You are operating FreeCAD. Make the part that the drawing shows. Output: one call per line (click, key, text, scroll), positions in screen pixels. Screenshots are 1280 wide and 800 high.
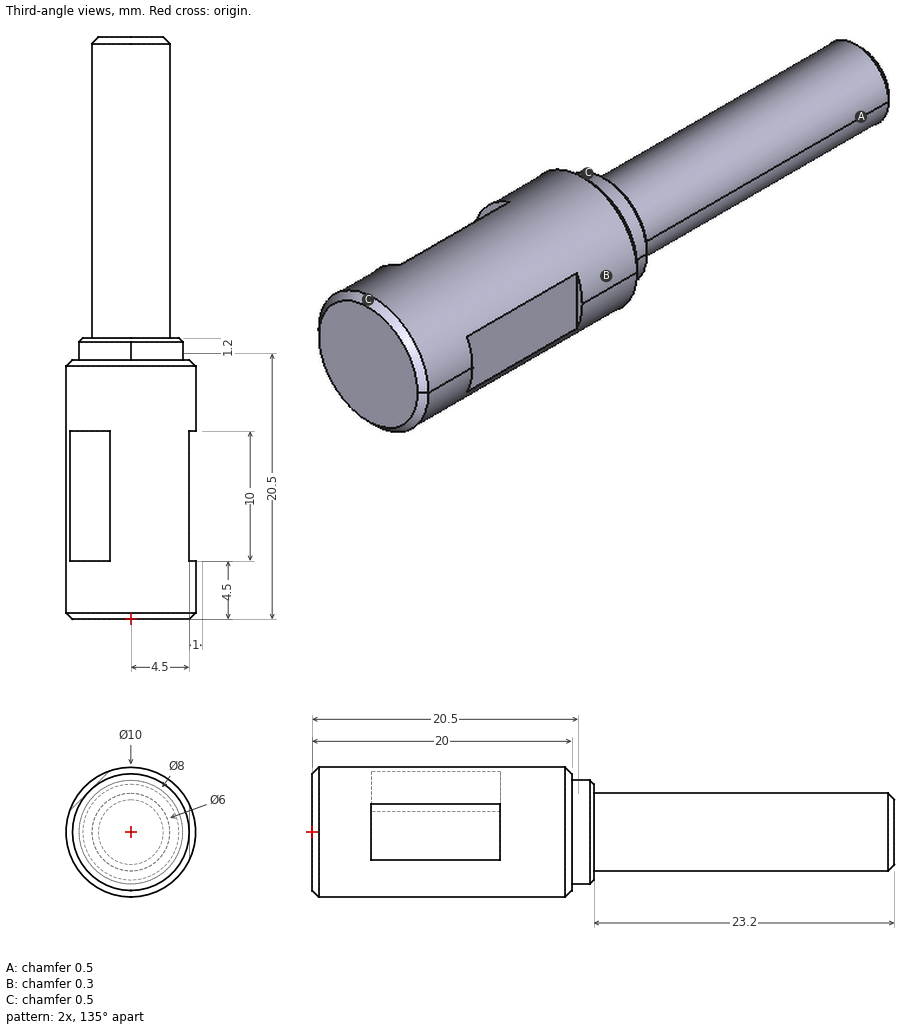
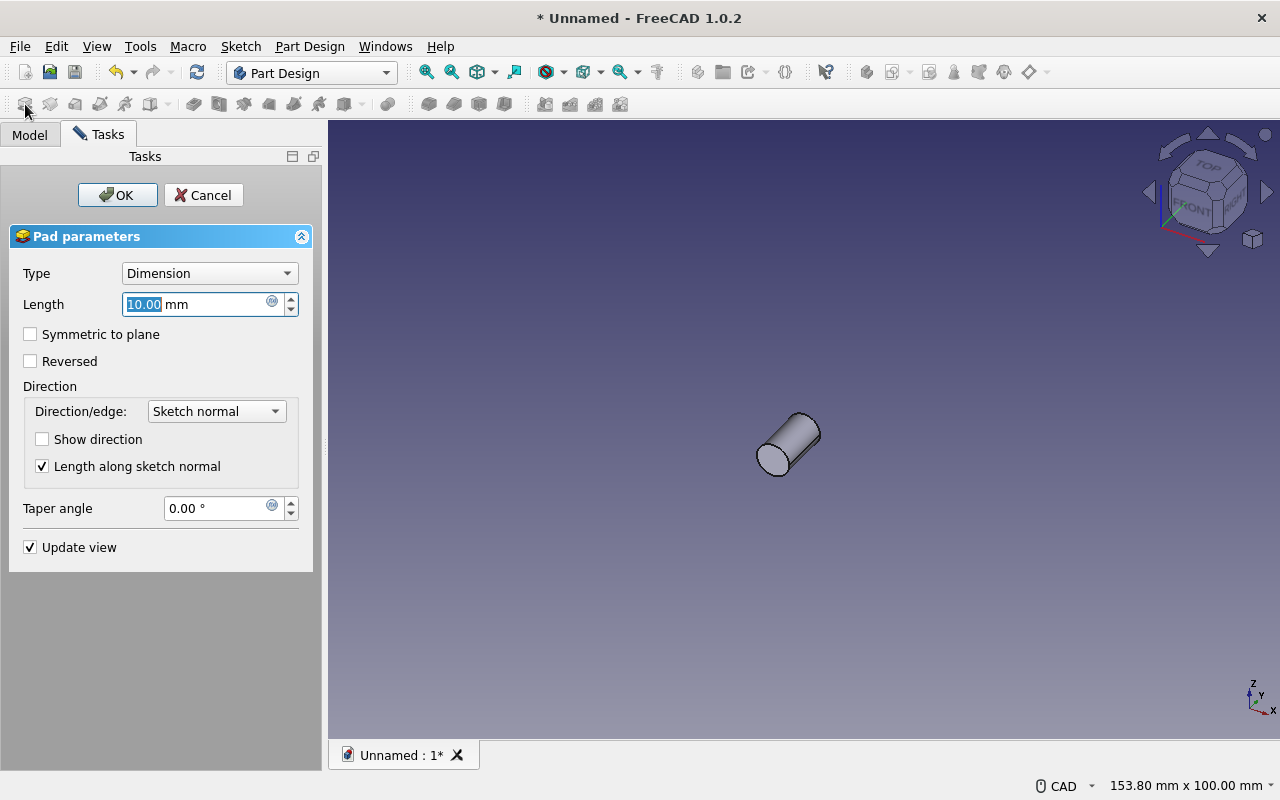
text(20.5)
key(Tab)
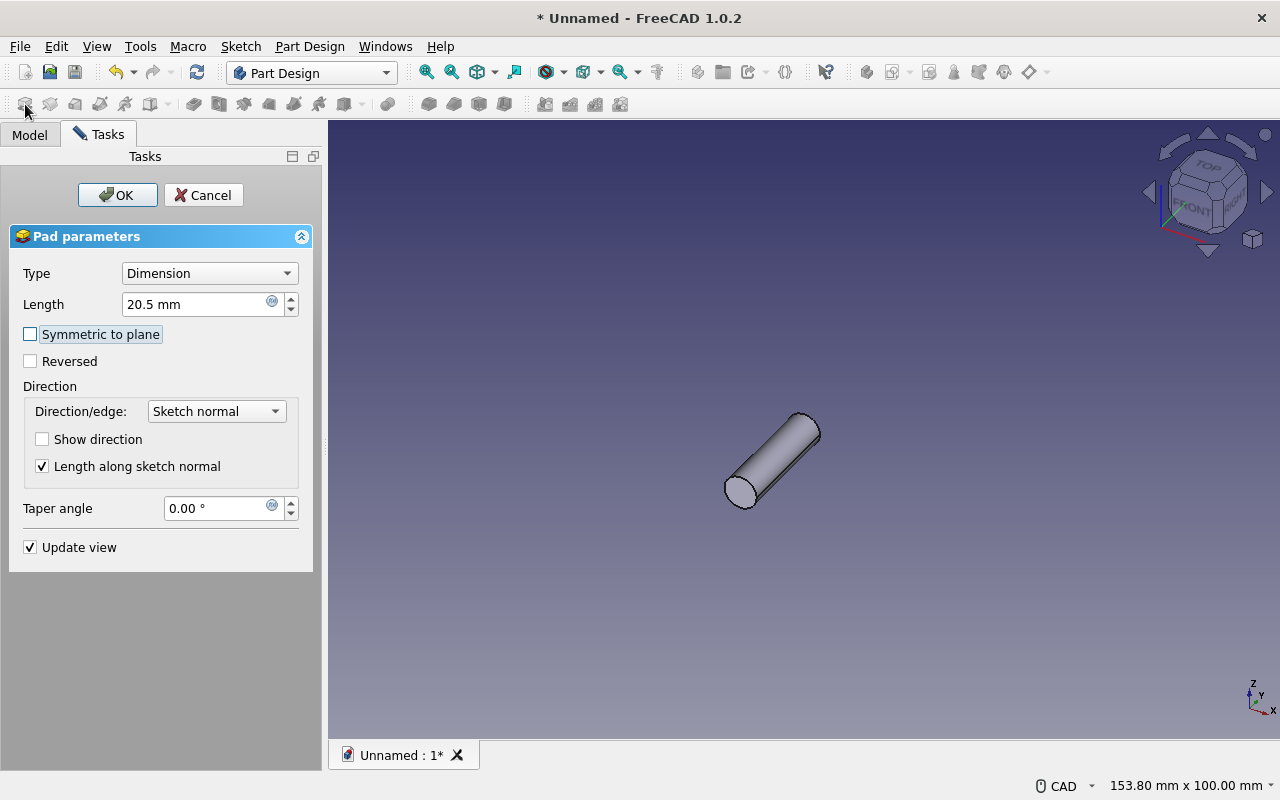
click(31, 361)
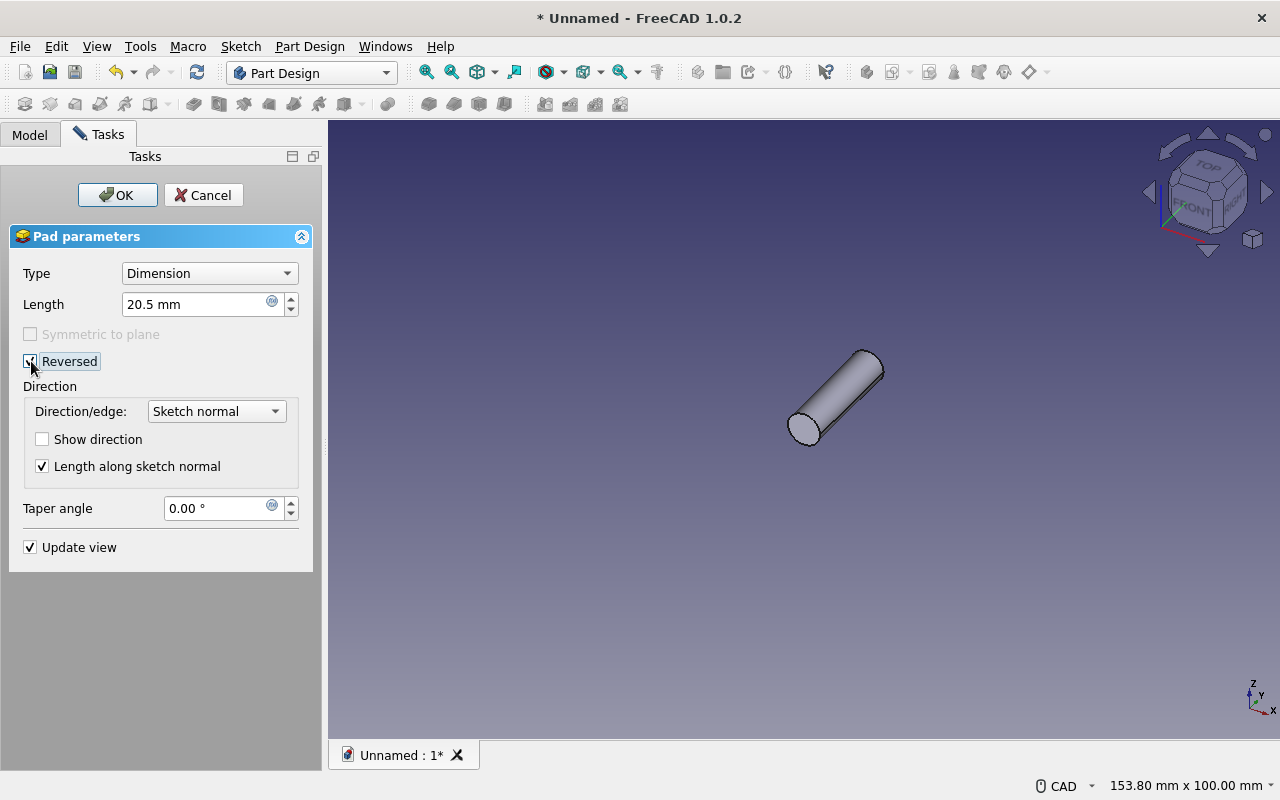
click(118, 195)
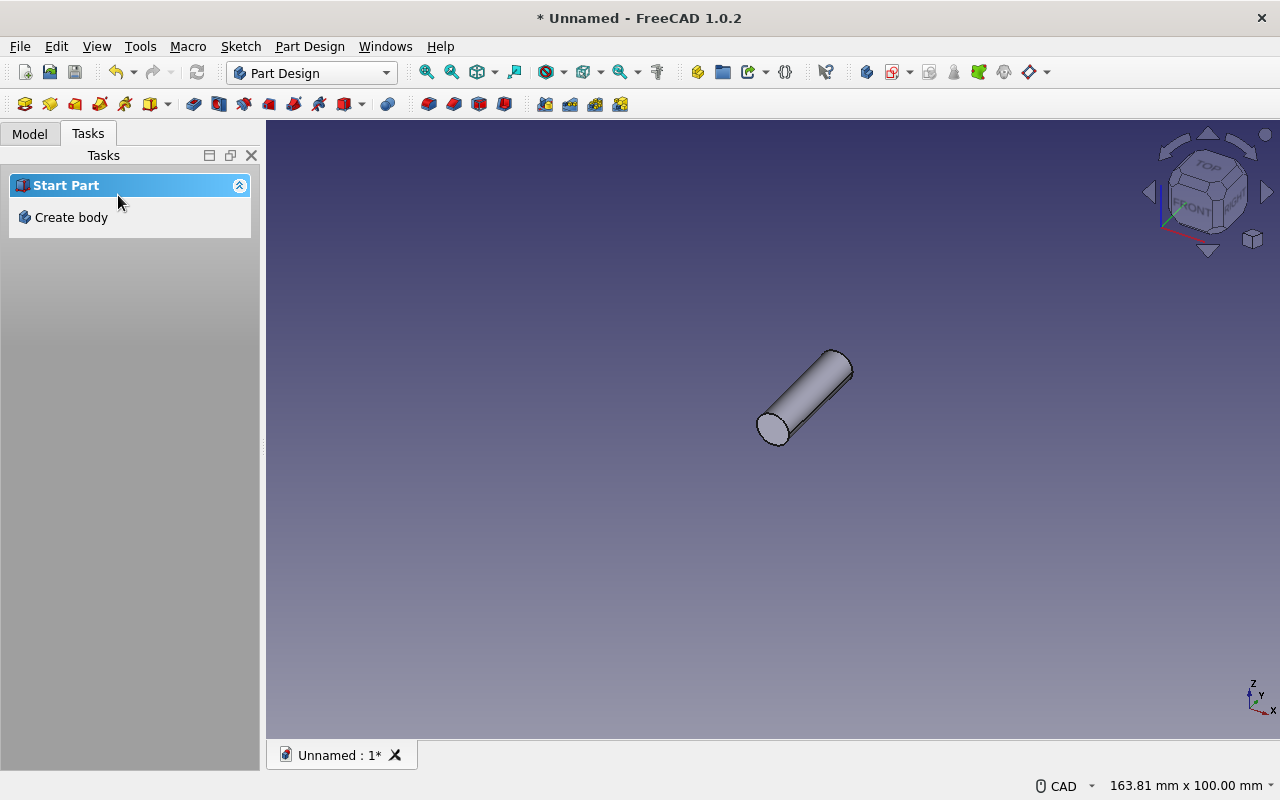
click(427, 72)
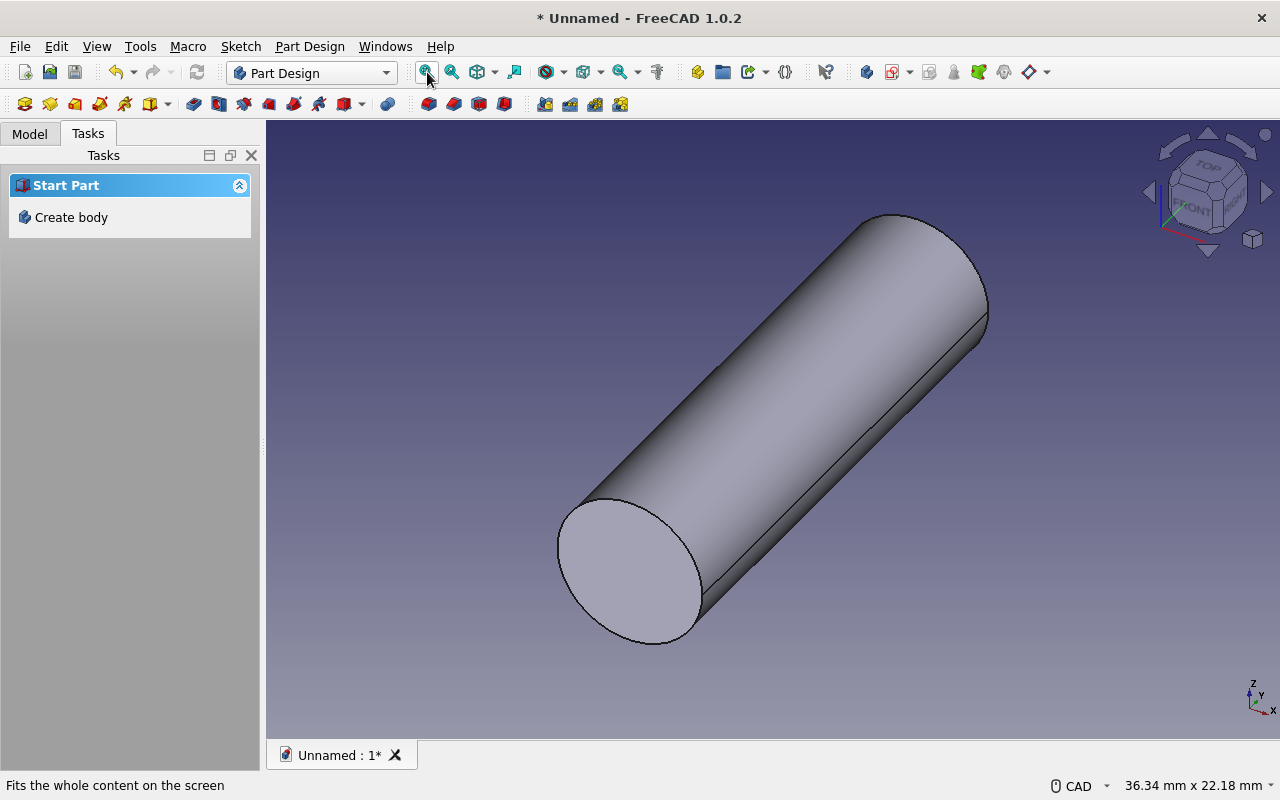
key(4)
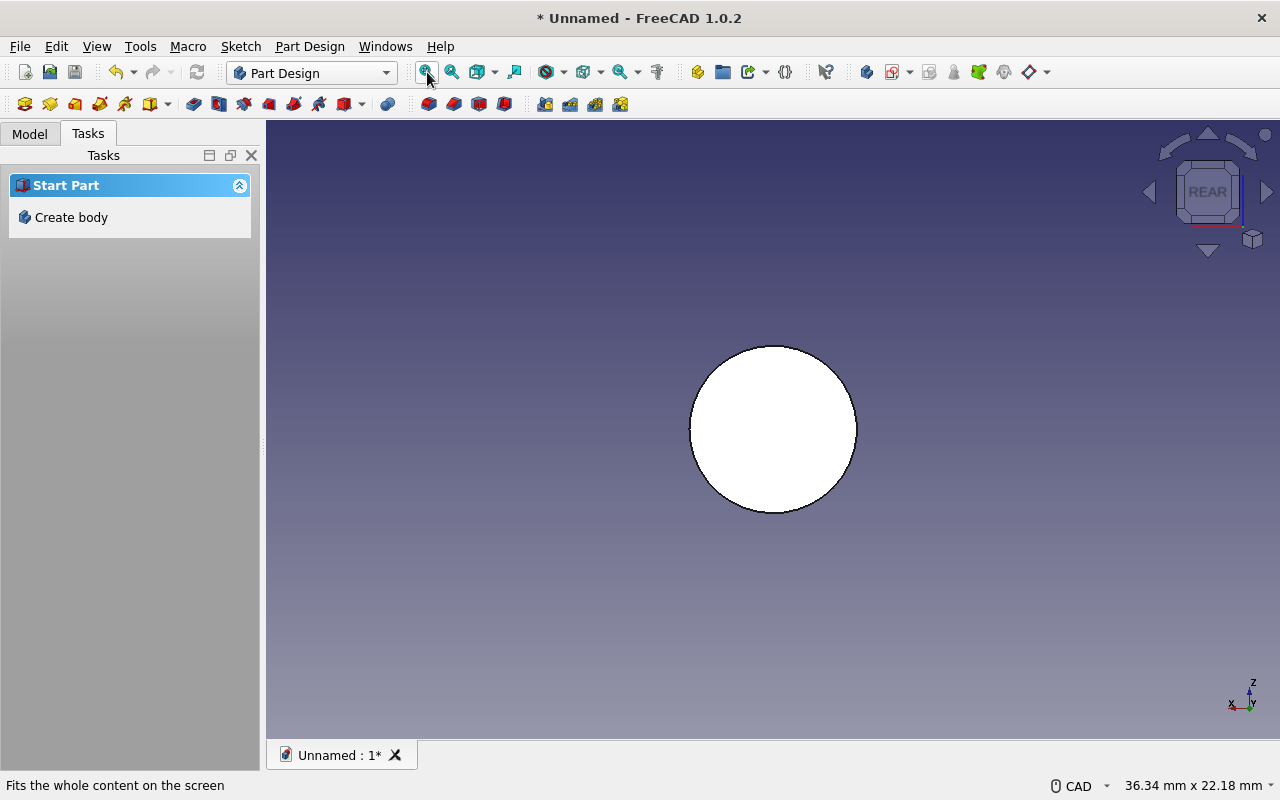
click(427, 72)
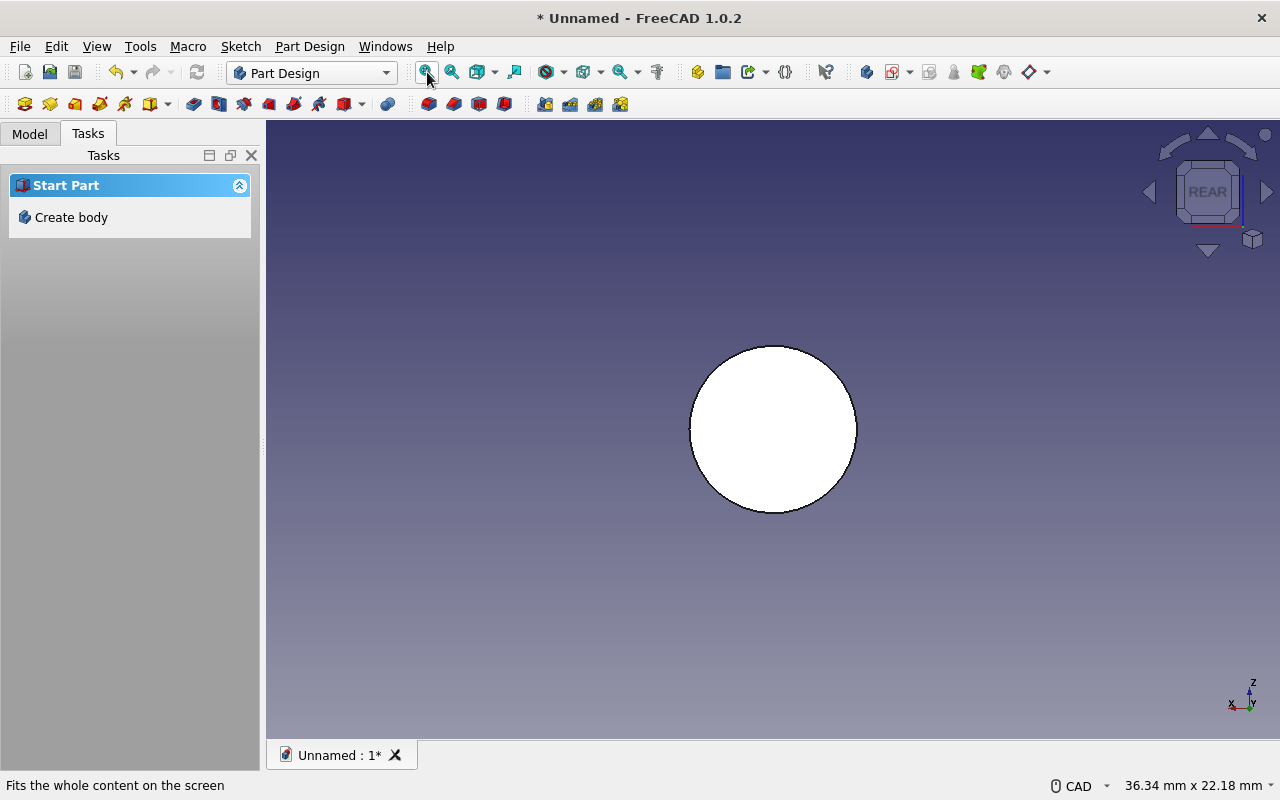
click(773, 429)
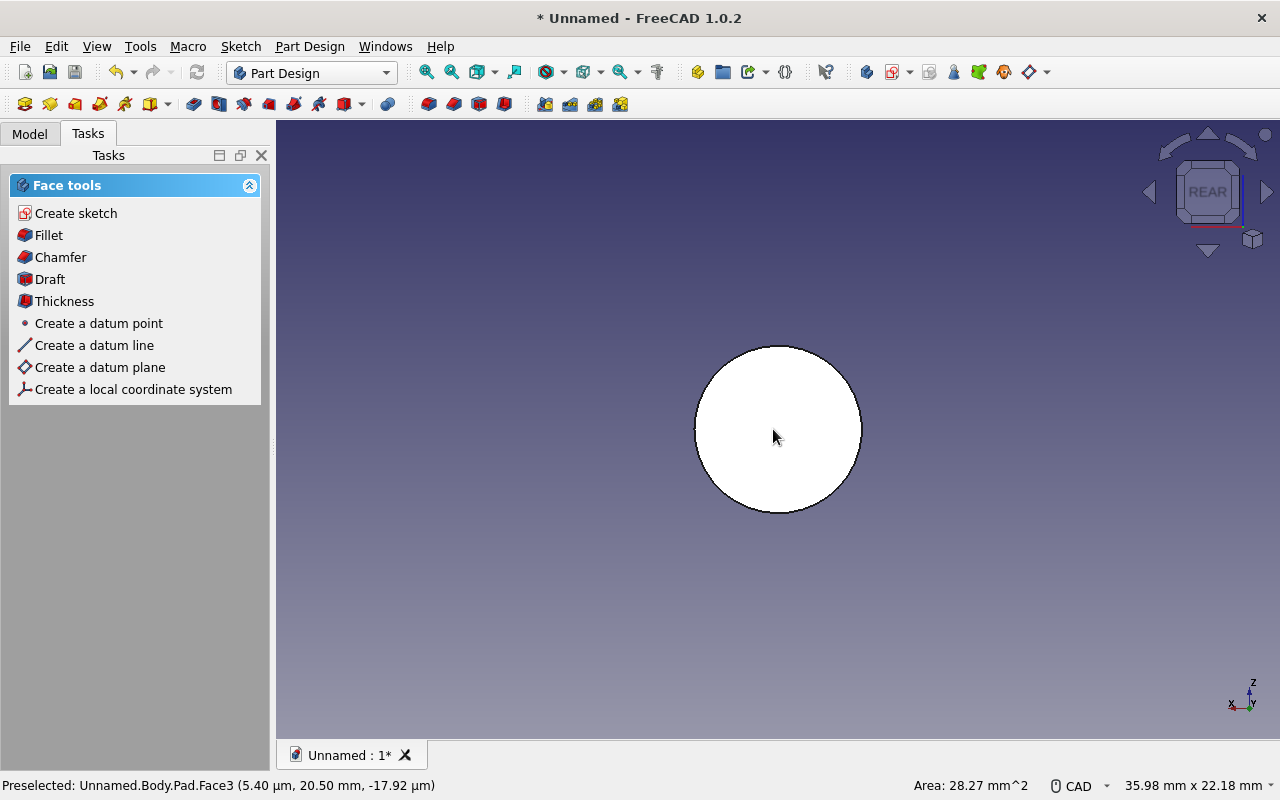
click(892, 72)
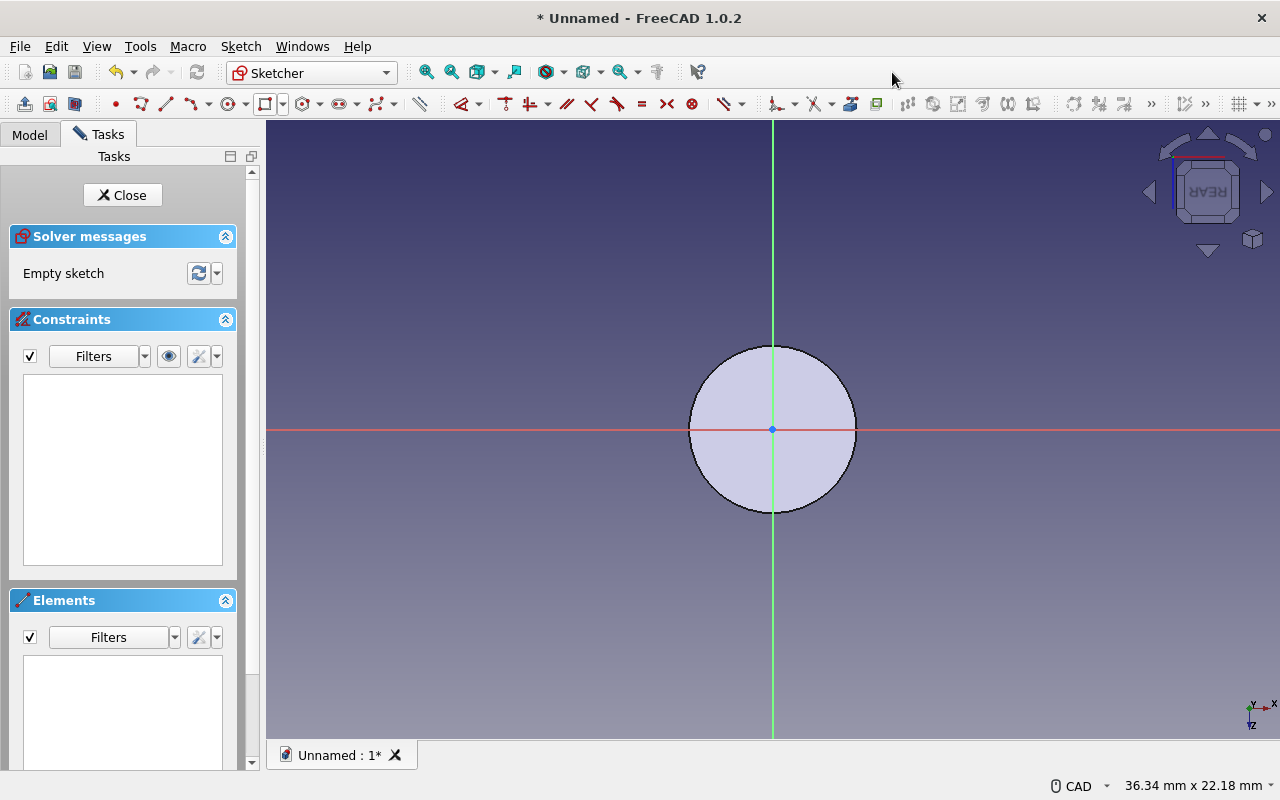
scroll(856, 429, up, 3)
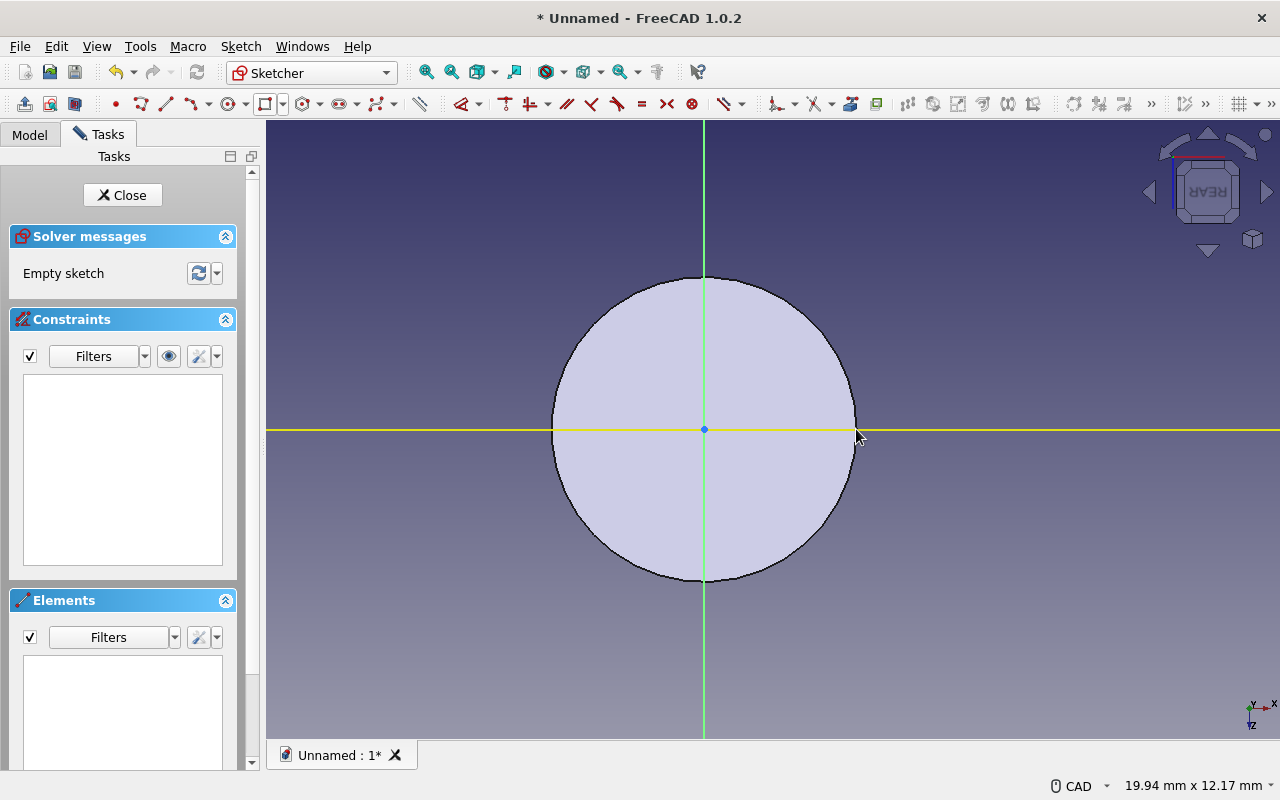
click(228, 104)